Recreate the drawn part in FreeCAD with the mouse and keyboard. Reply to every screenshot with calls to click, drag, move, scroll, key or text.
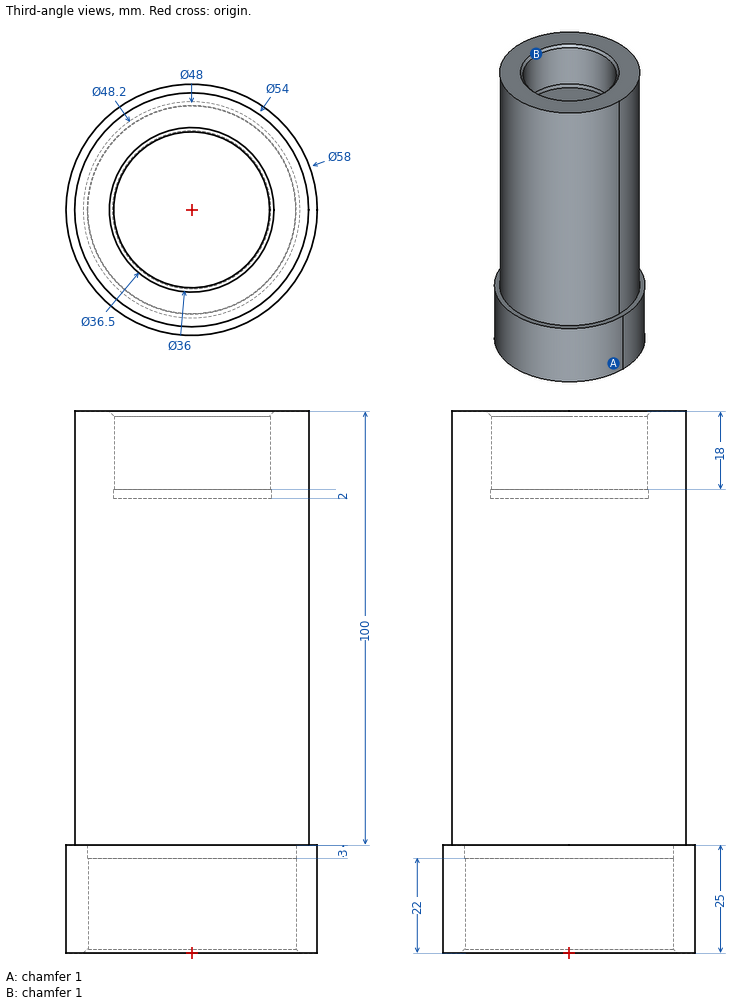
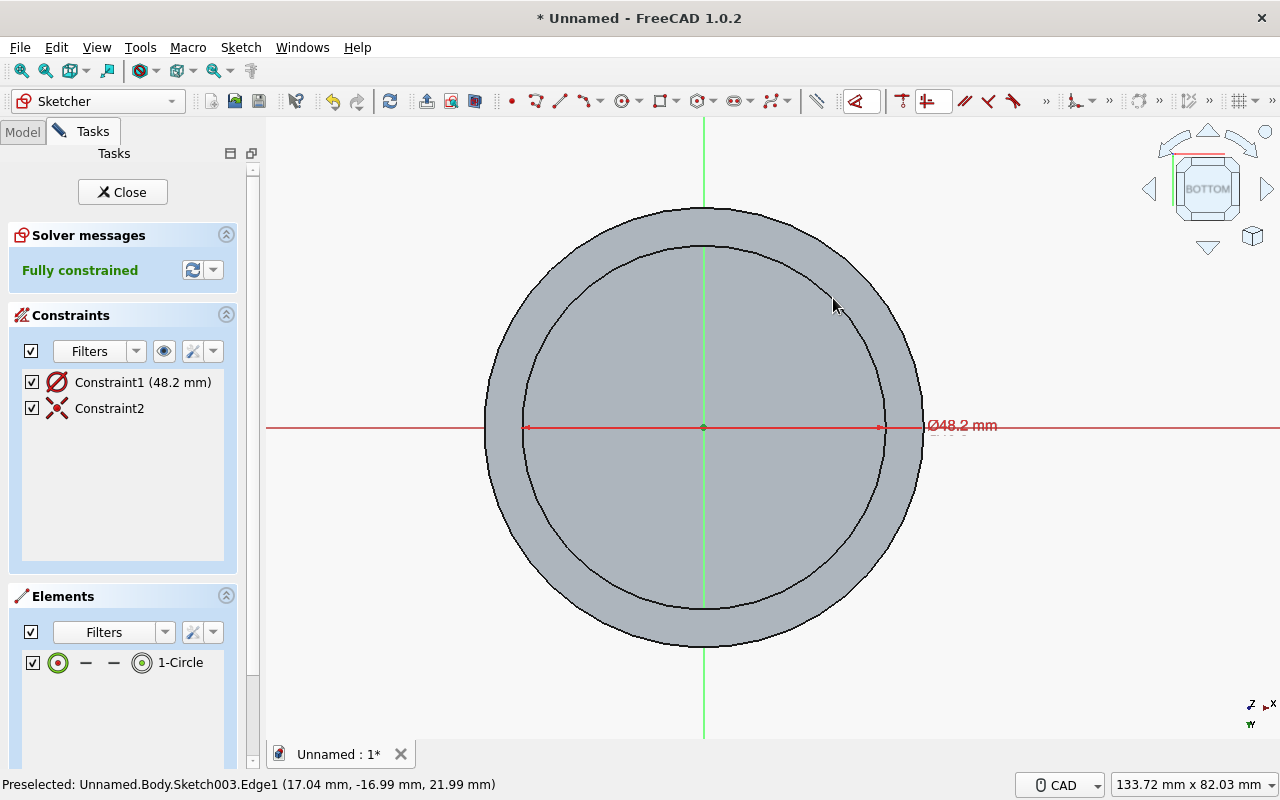
click(123, 192)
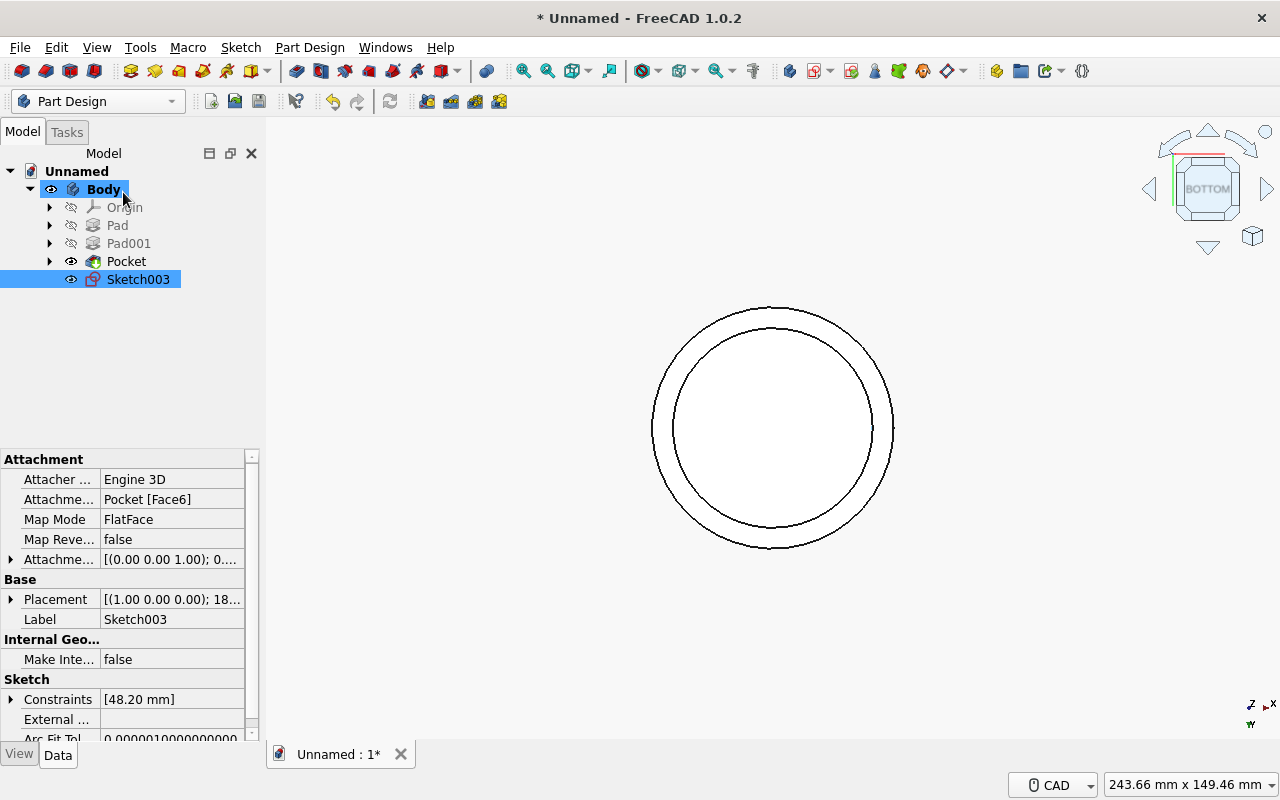
click(298, 72)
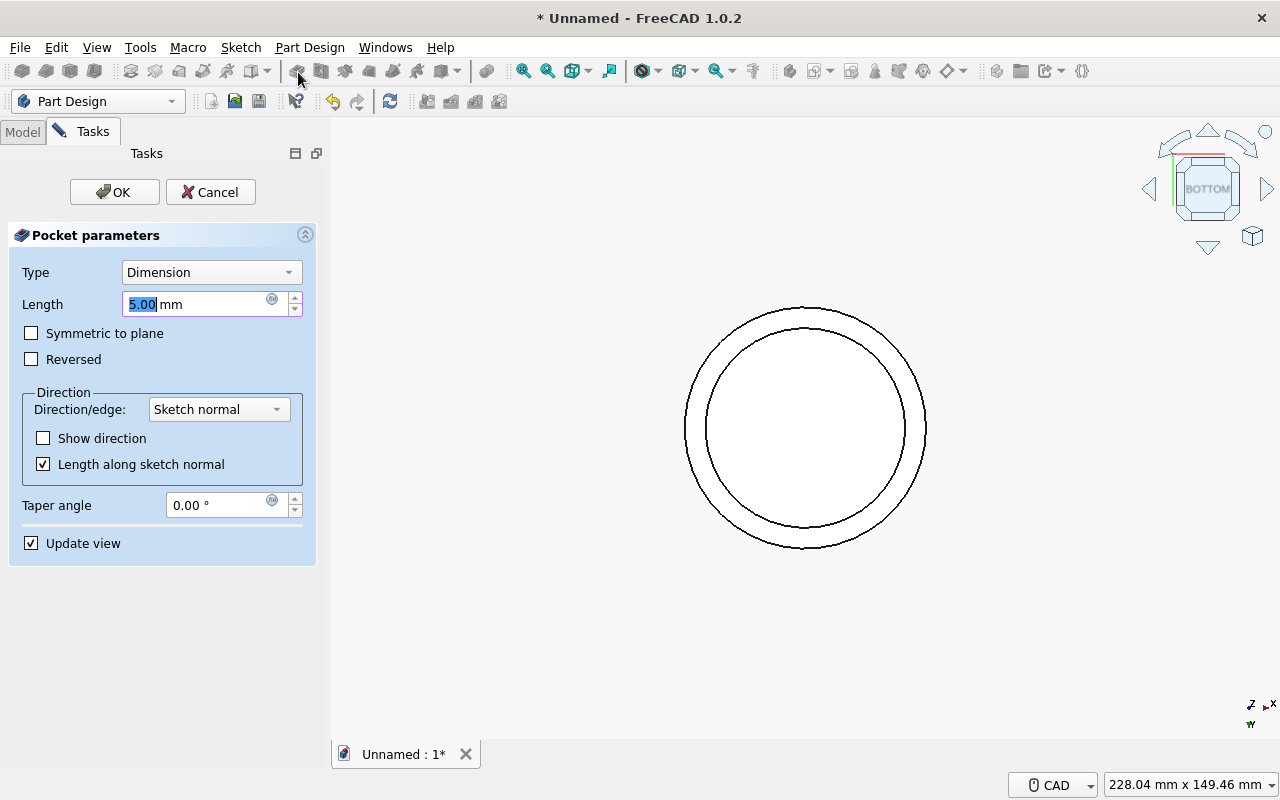
text(3)
key(Tab)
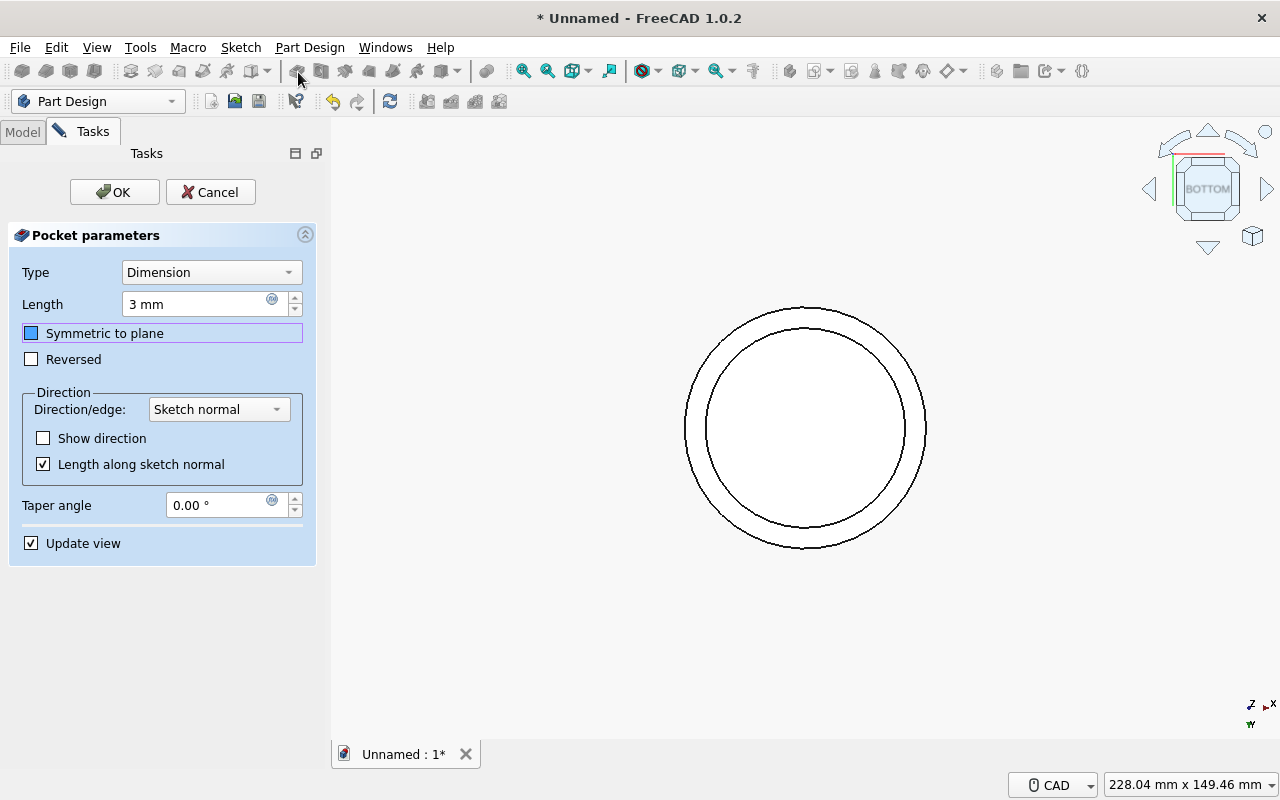
click(115, 192)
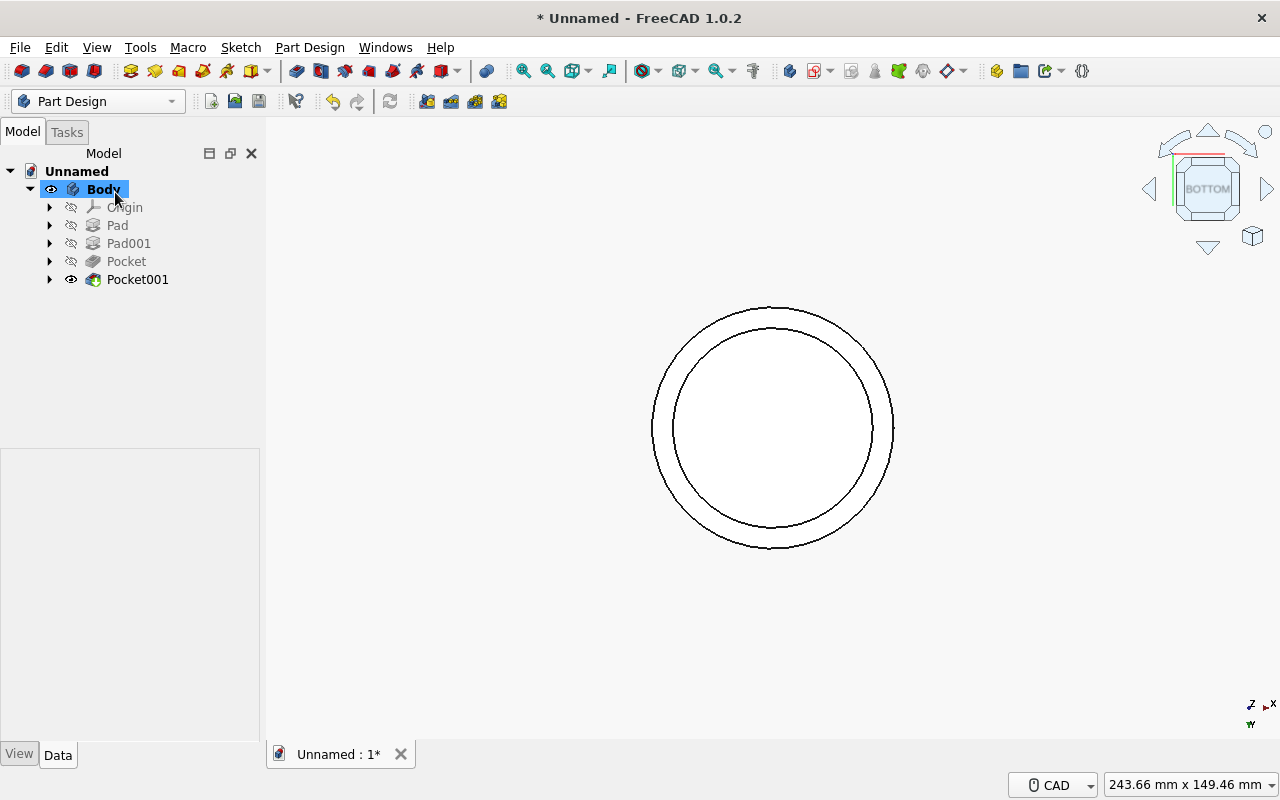
click(524, 72)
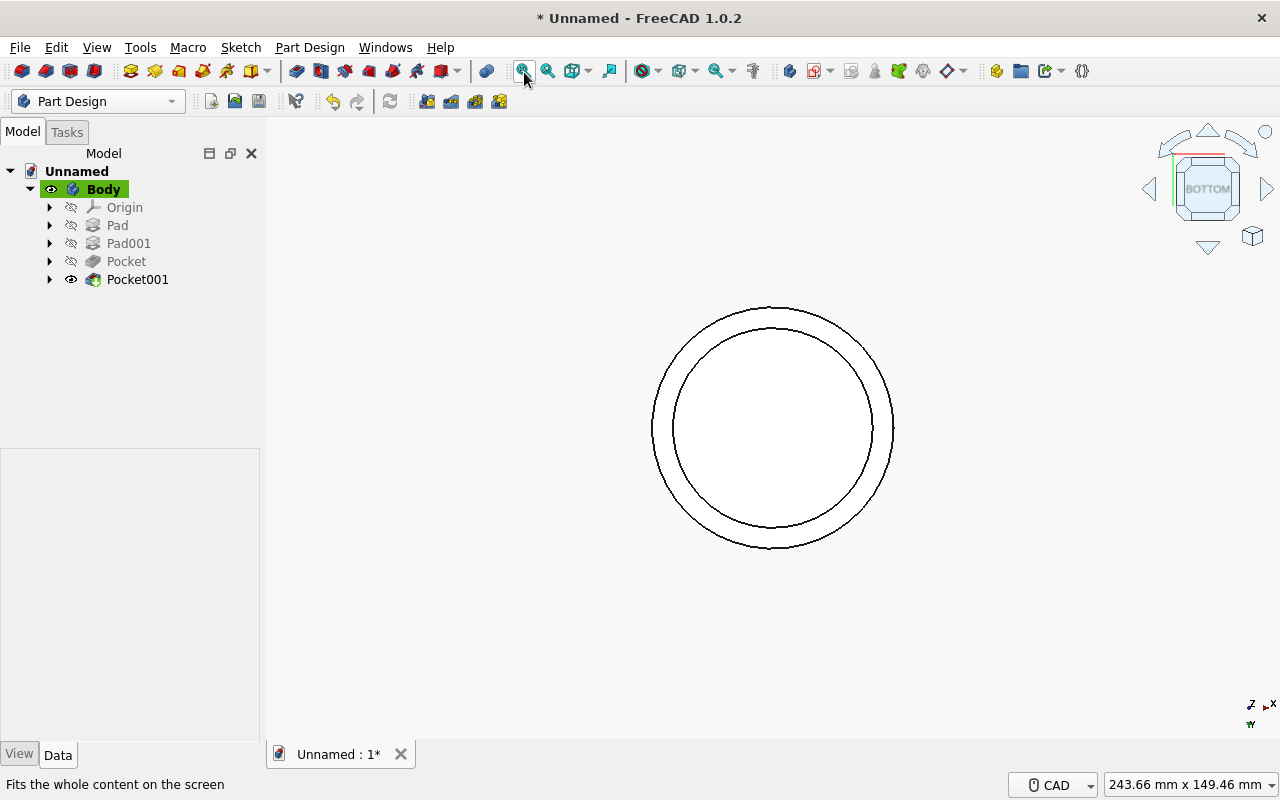
click(673, 427)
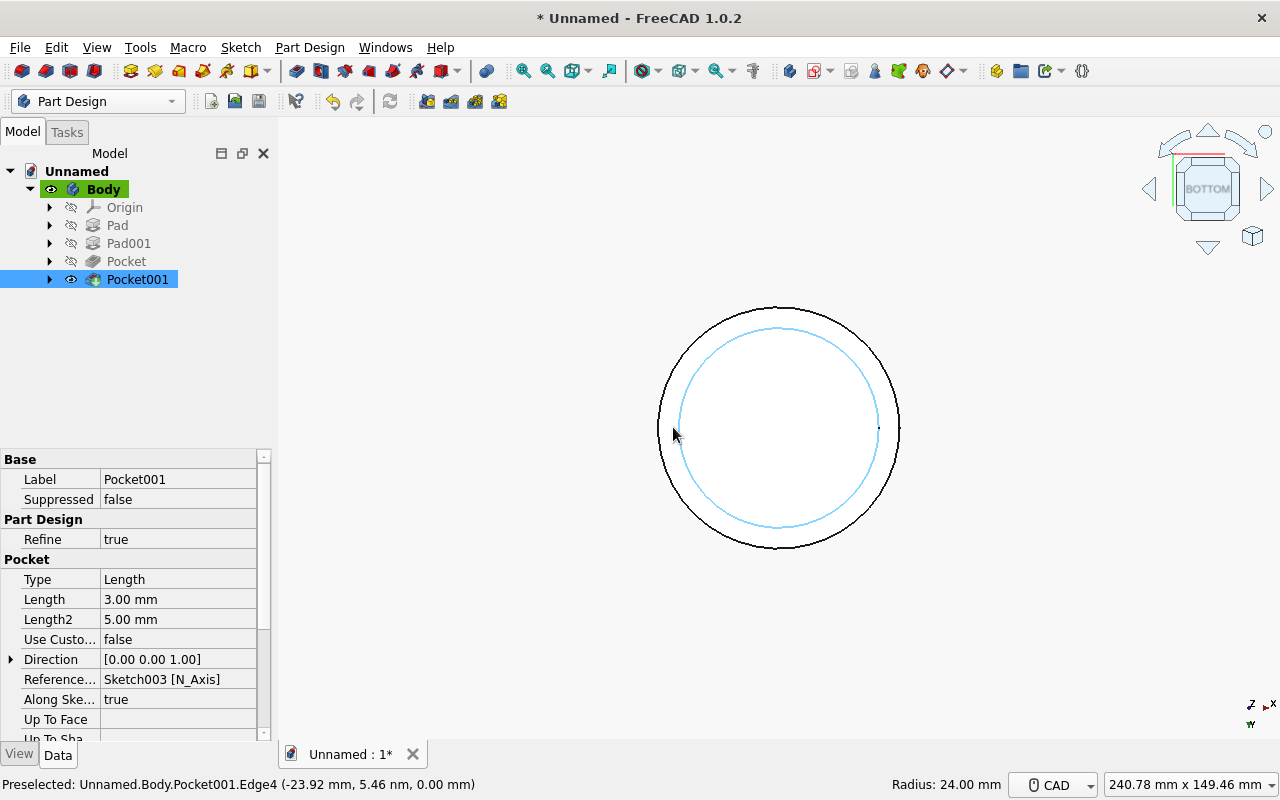
click(46, 72)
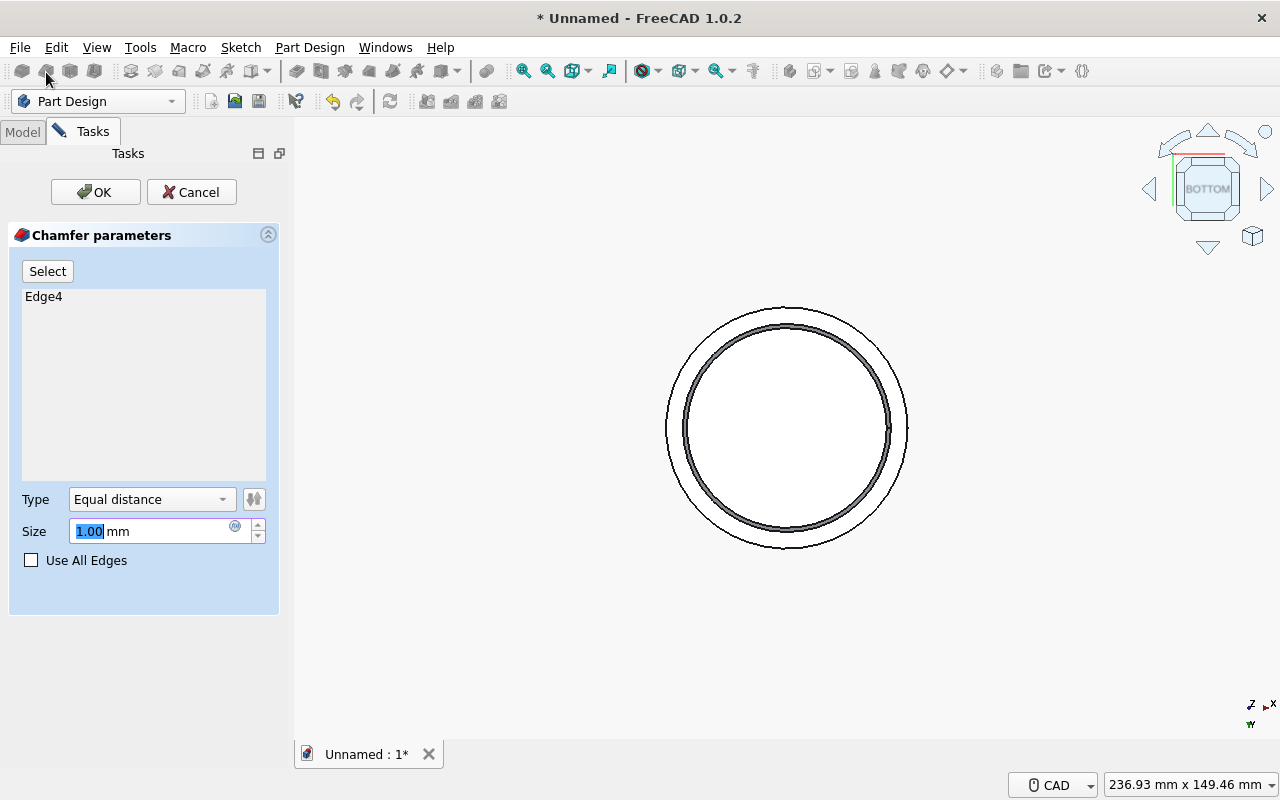
text(1)
key(Tab)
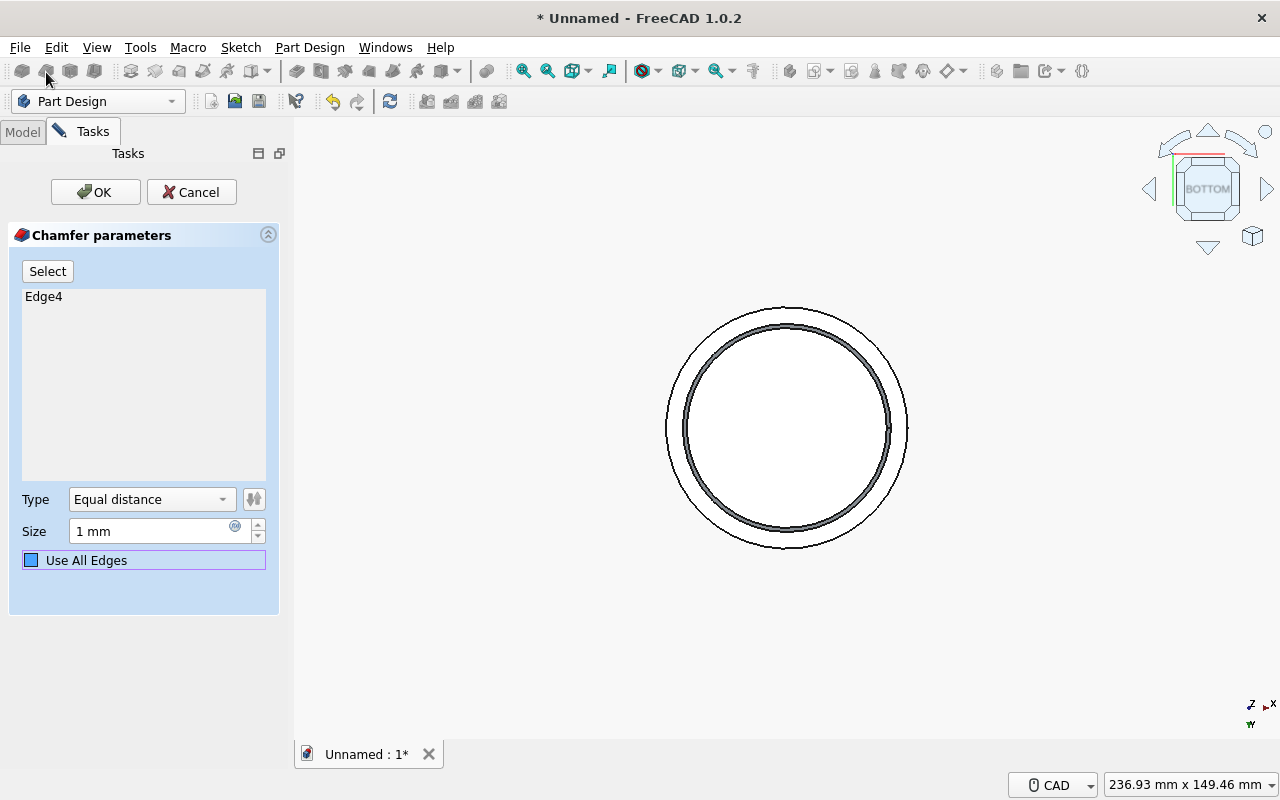
click(96, 192)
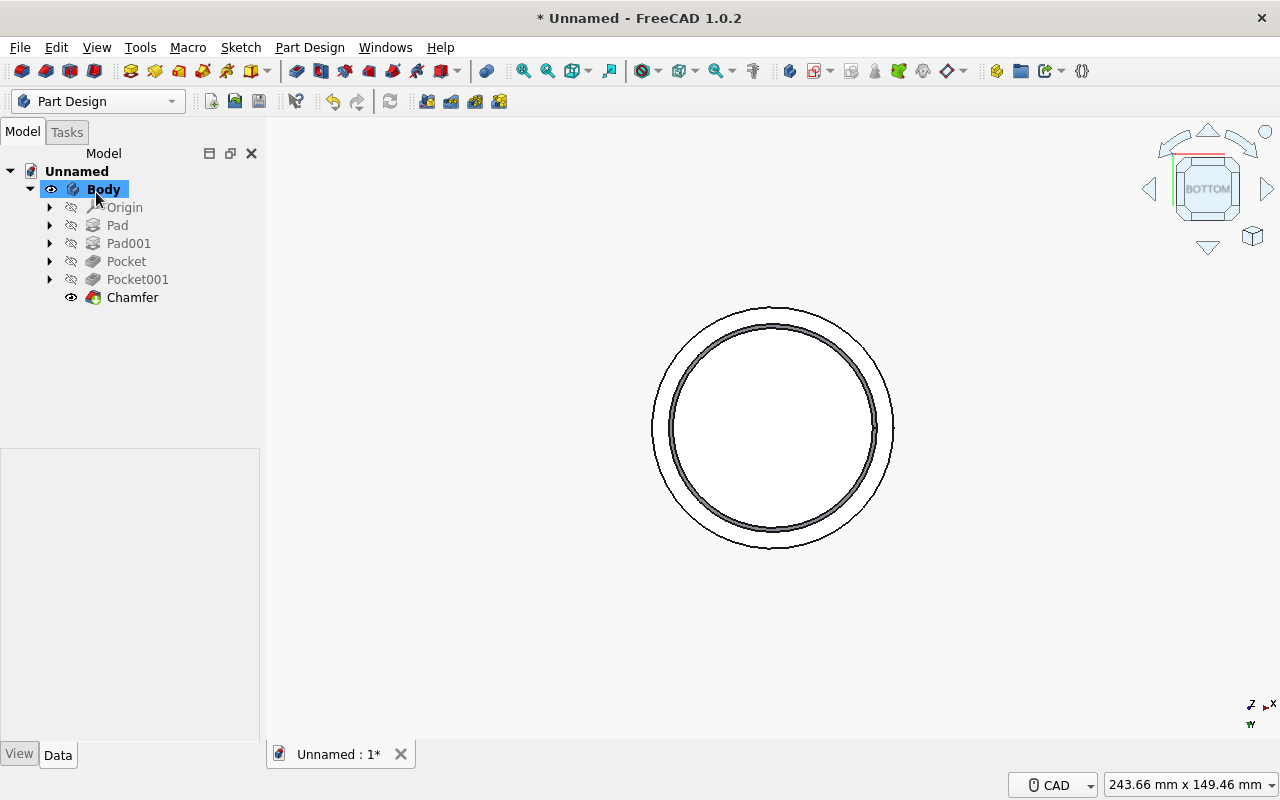
click(524, 72)